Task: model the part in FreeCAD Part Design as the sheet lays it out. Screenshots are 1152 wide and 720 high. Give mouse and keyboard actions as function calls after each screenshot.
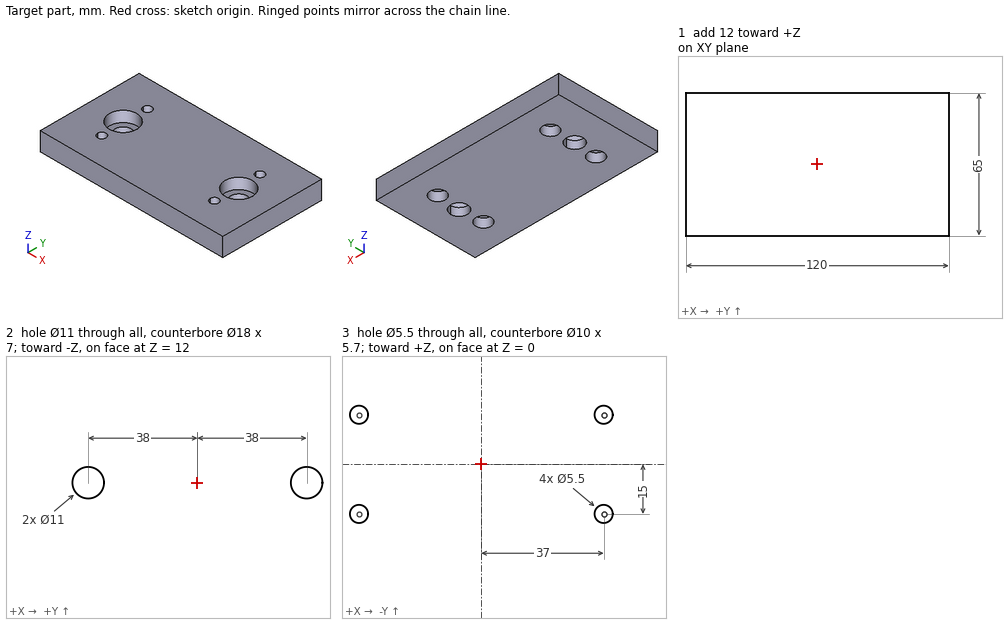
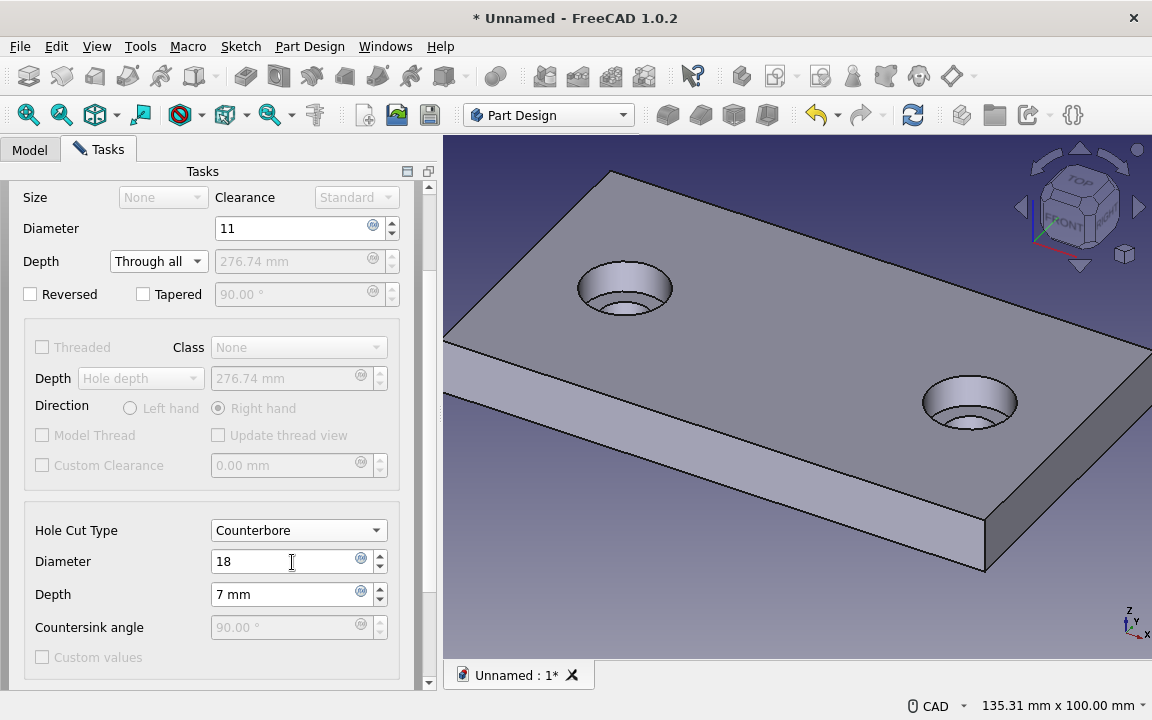
scroll(429, 436, up, 3)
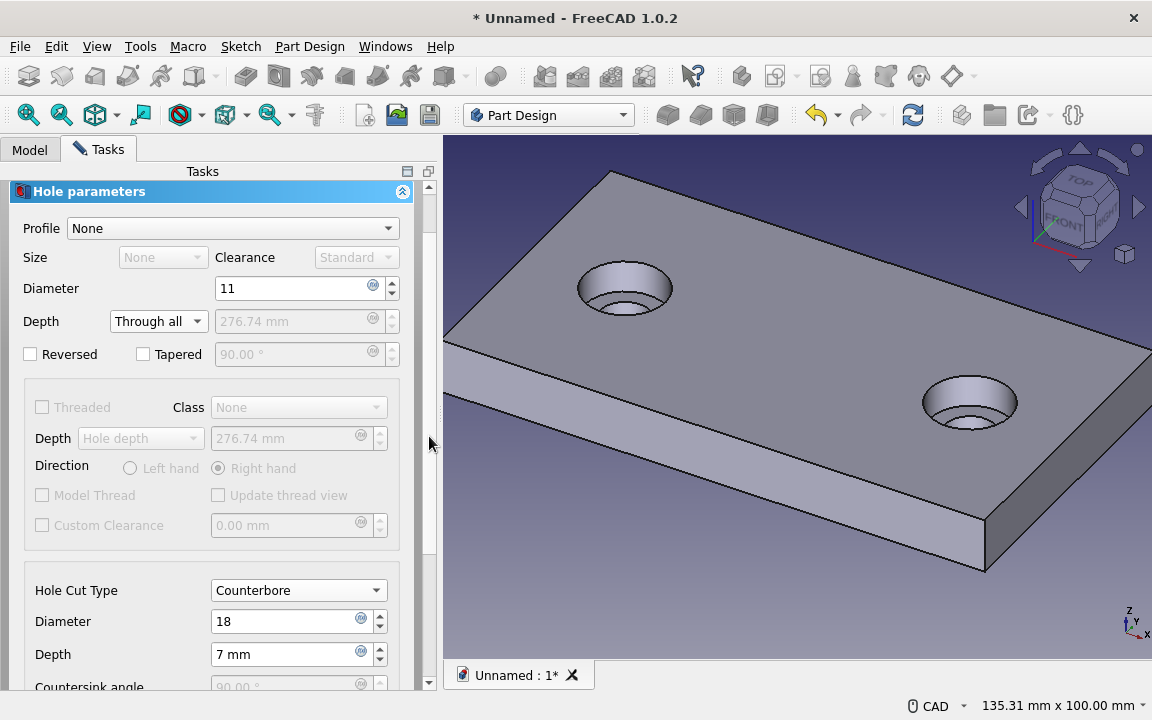
click(169, 210)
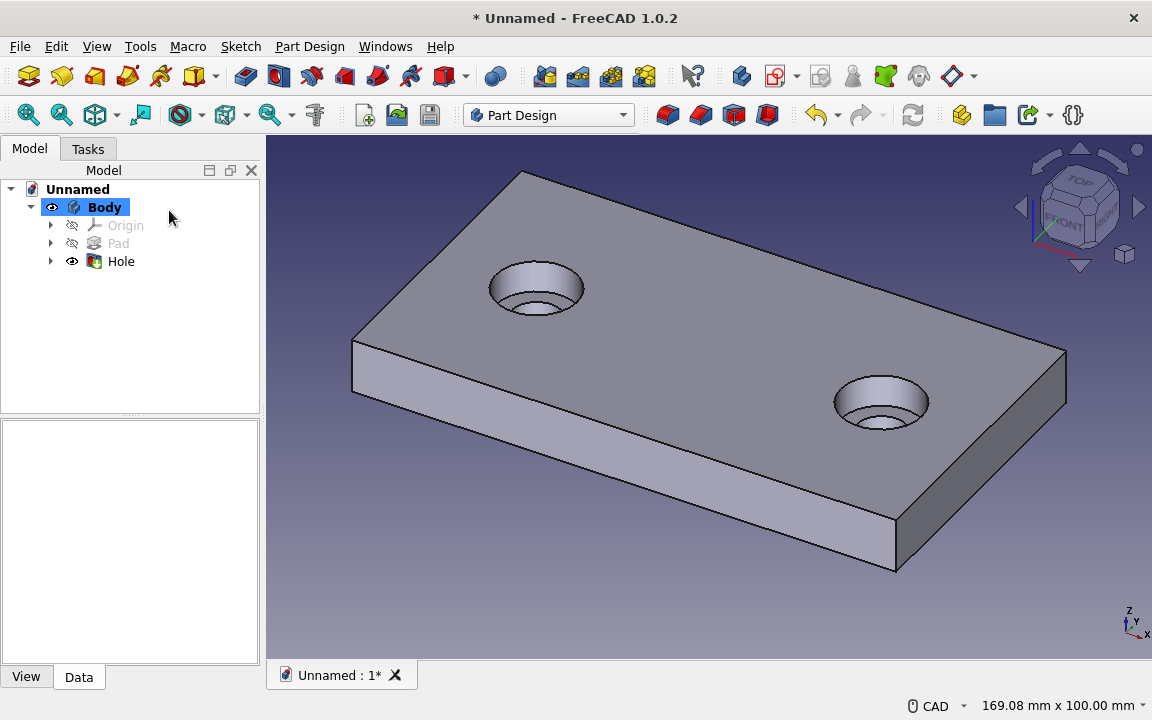
key(5)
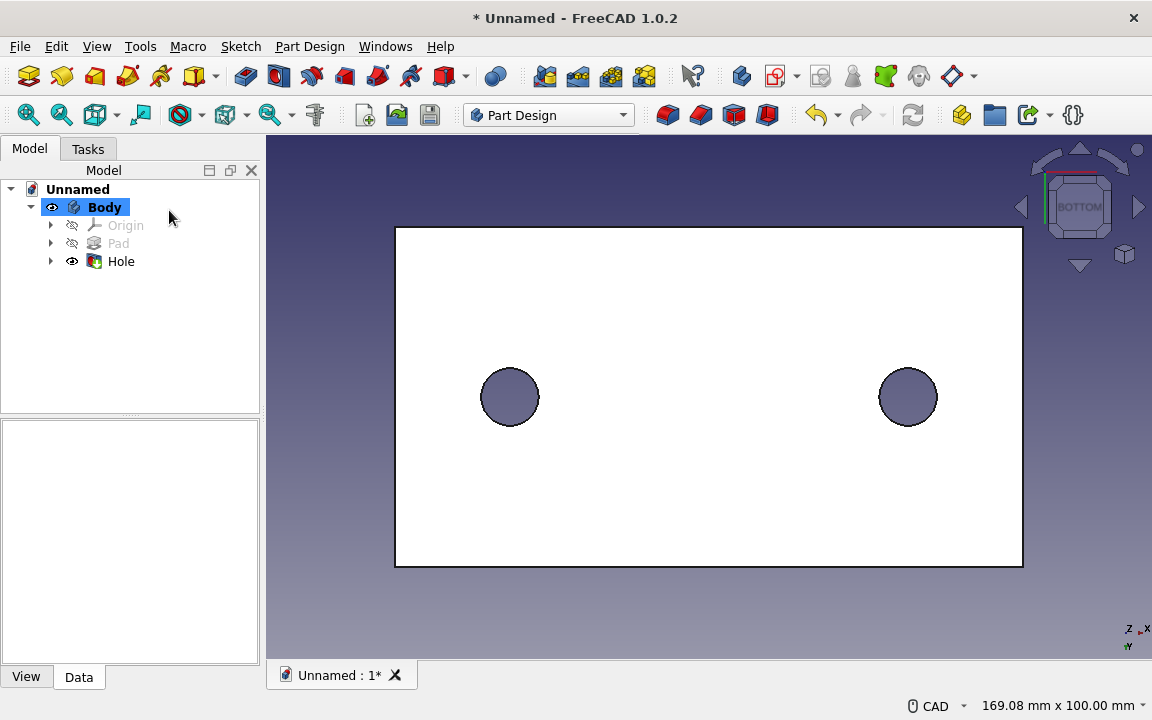
click(709, 396)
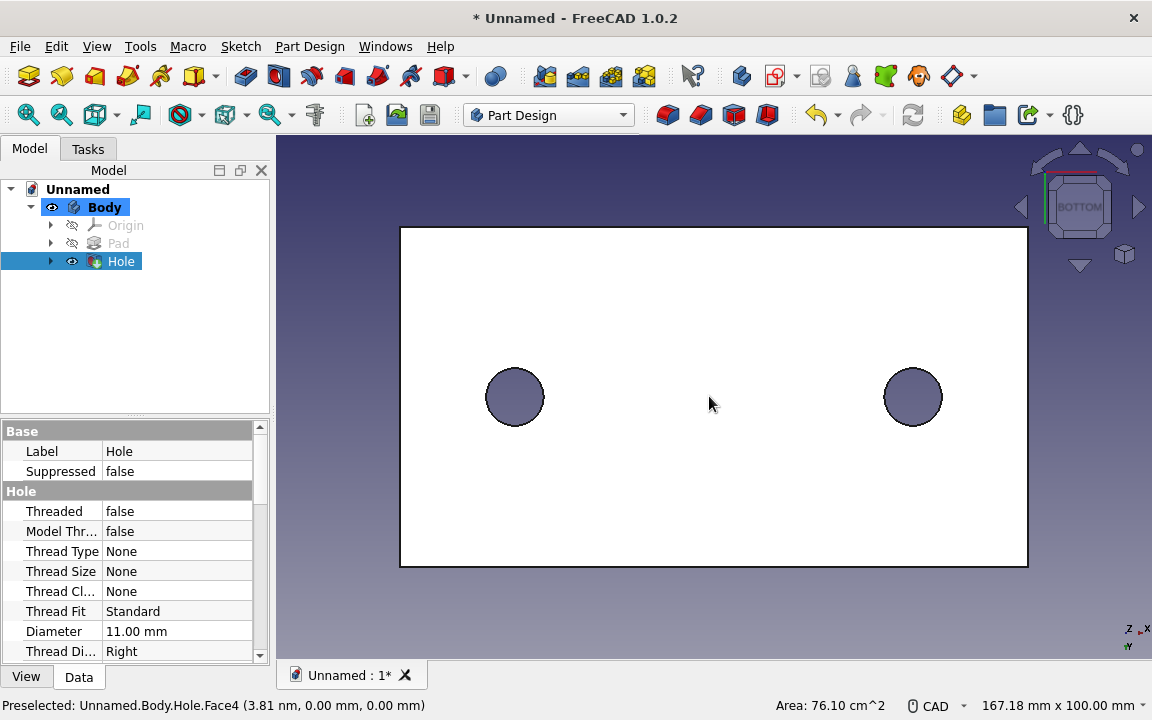
click(774, 76)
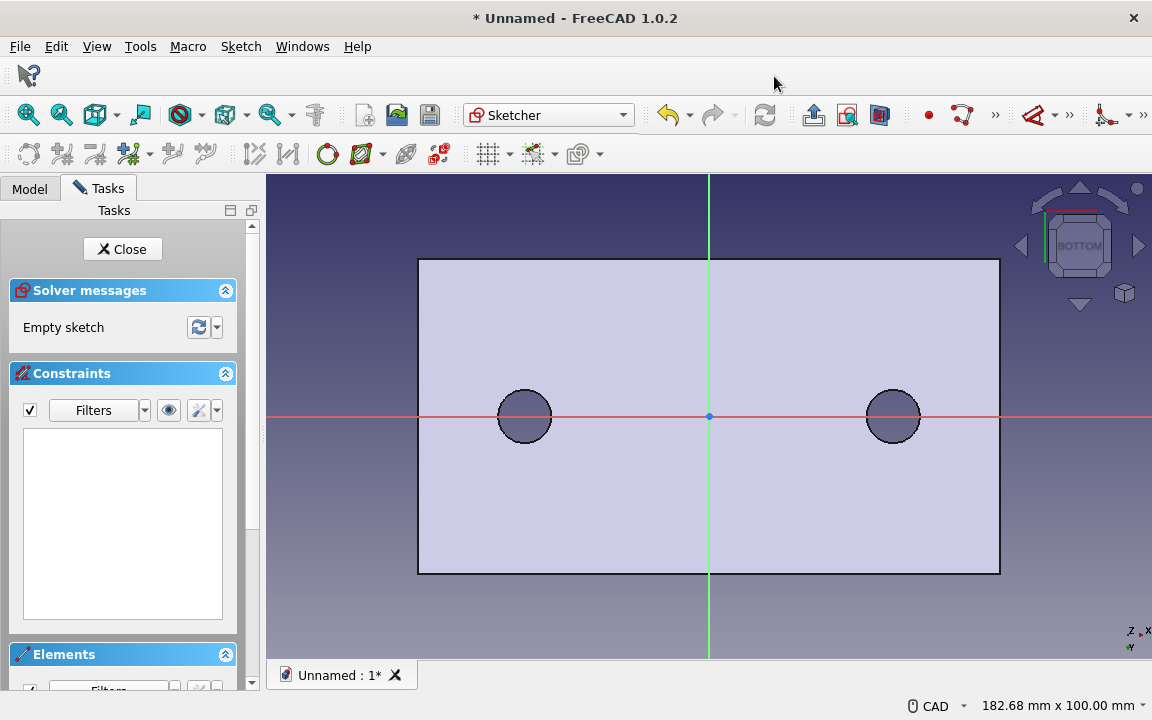
key(g)
key(c)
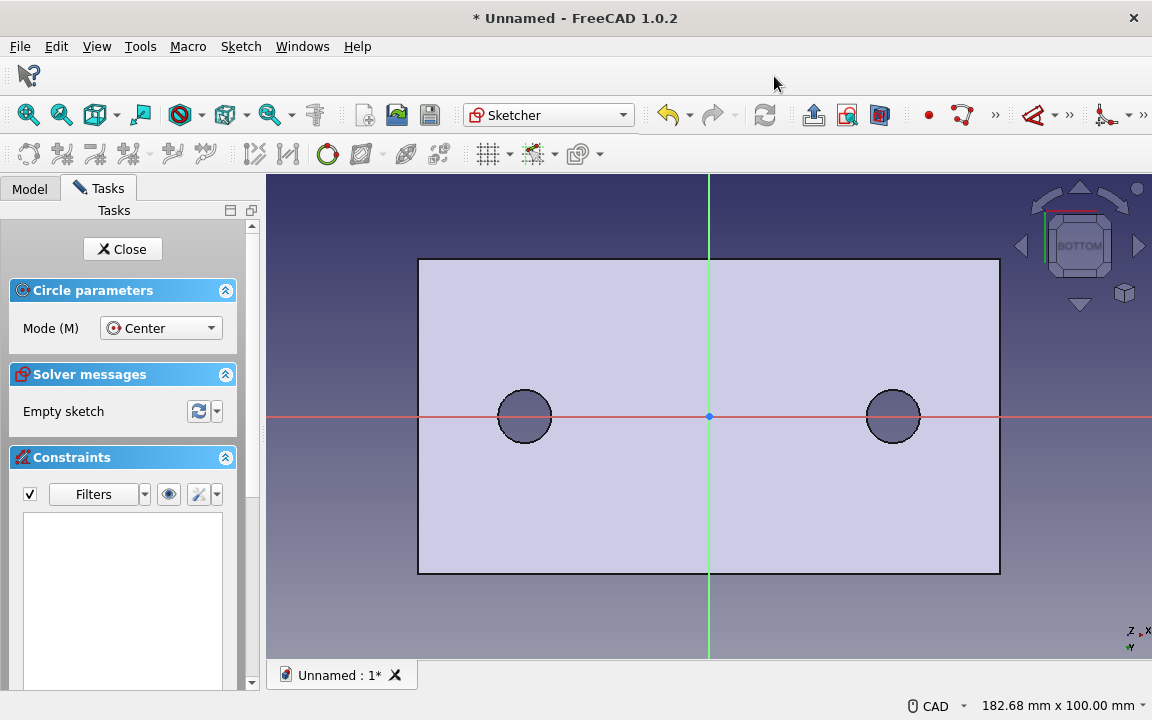
scroll(888, 489, up, 3)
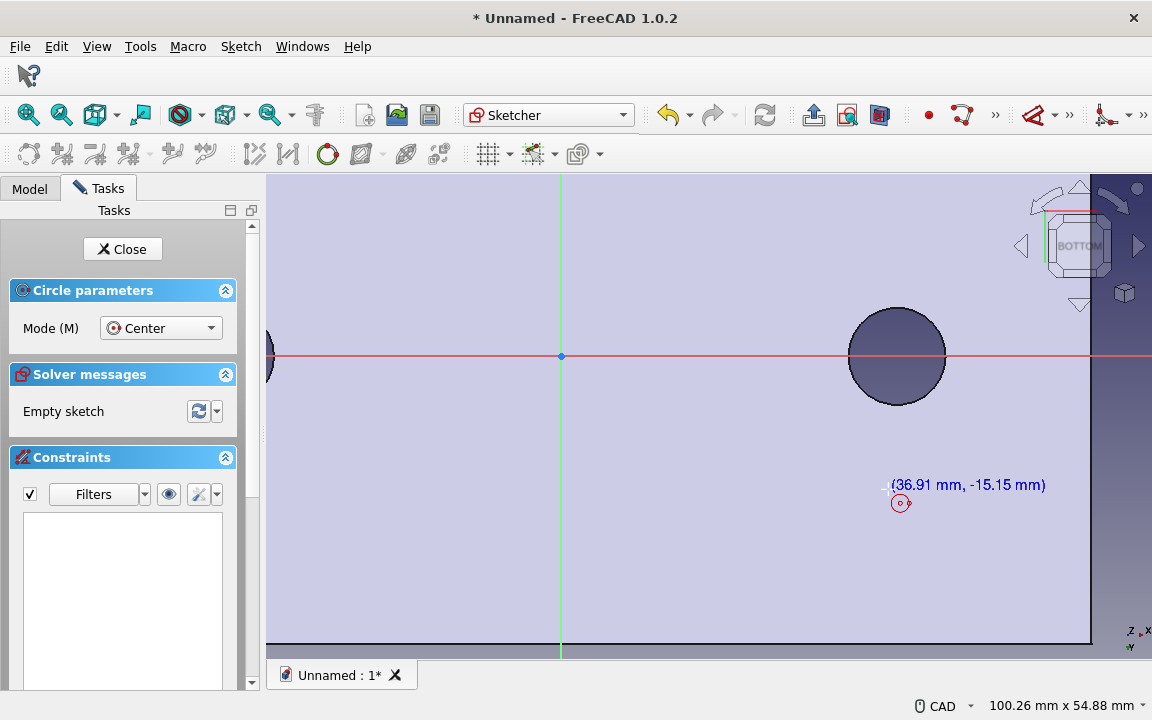
click(888, 489)
move(905, 472)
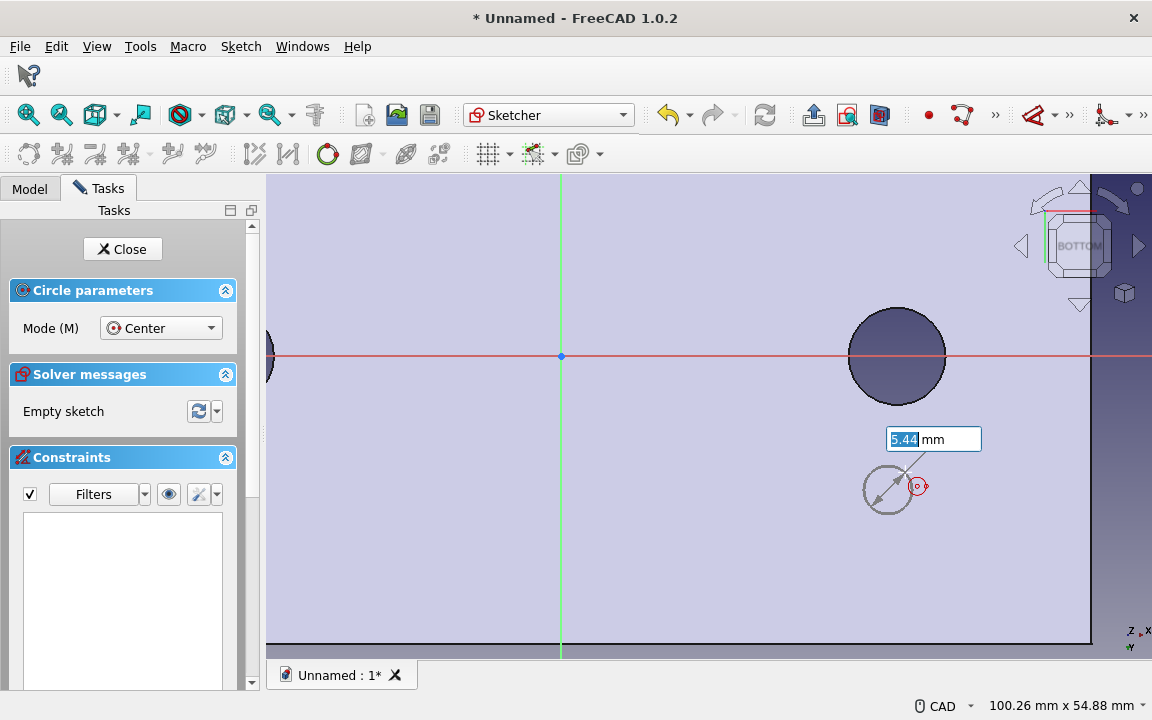
text(5.5)
key(Return)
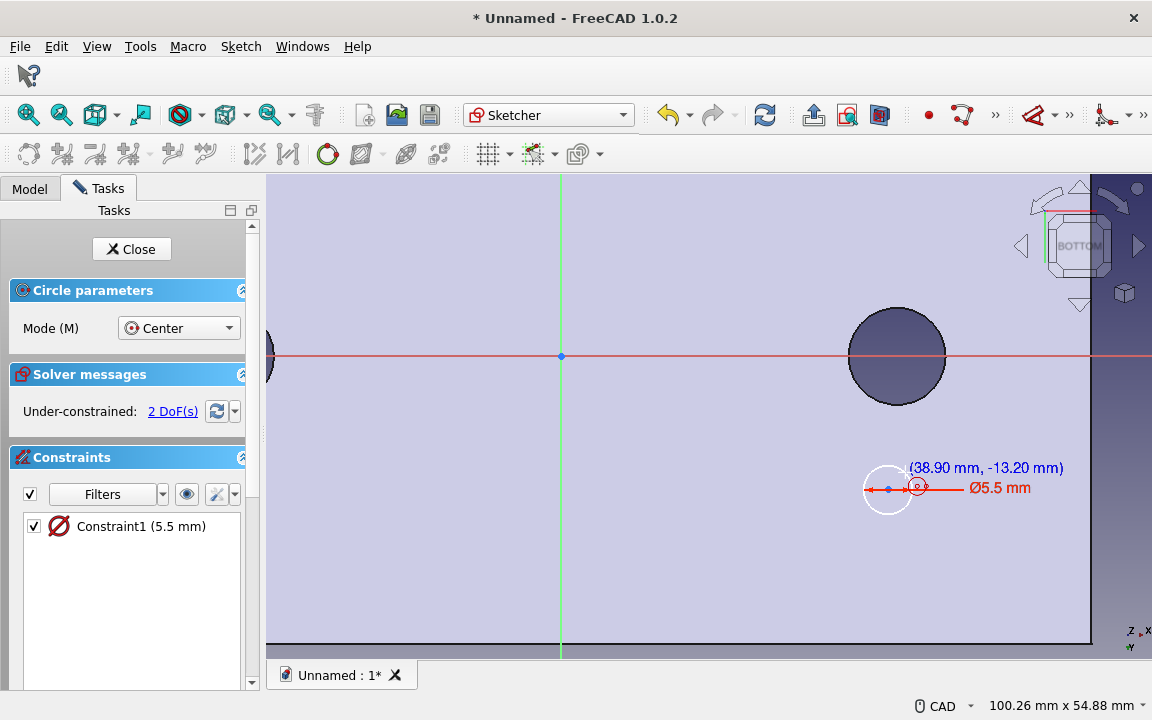
click(888, 224)
move(905, 207)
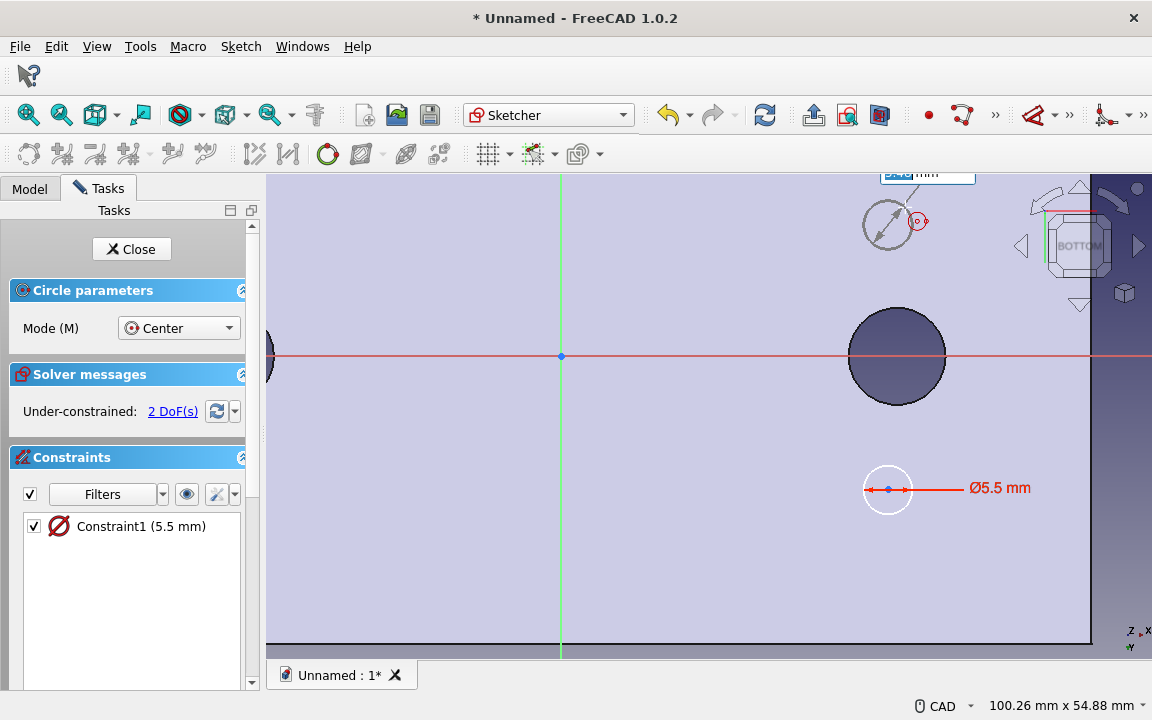
text(5.5)
key(Return)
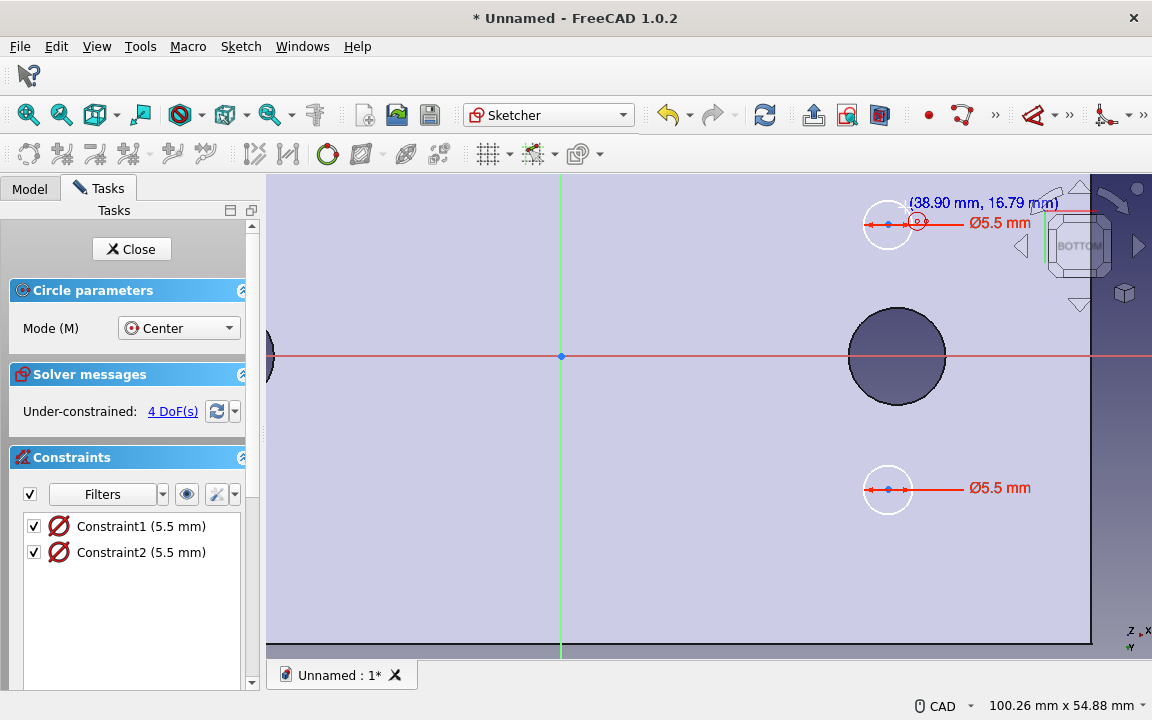
scroll(802, 539, down, 2)